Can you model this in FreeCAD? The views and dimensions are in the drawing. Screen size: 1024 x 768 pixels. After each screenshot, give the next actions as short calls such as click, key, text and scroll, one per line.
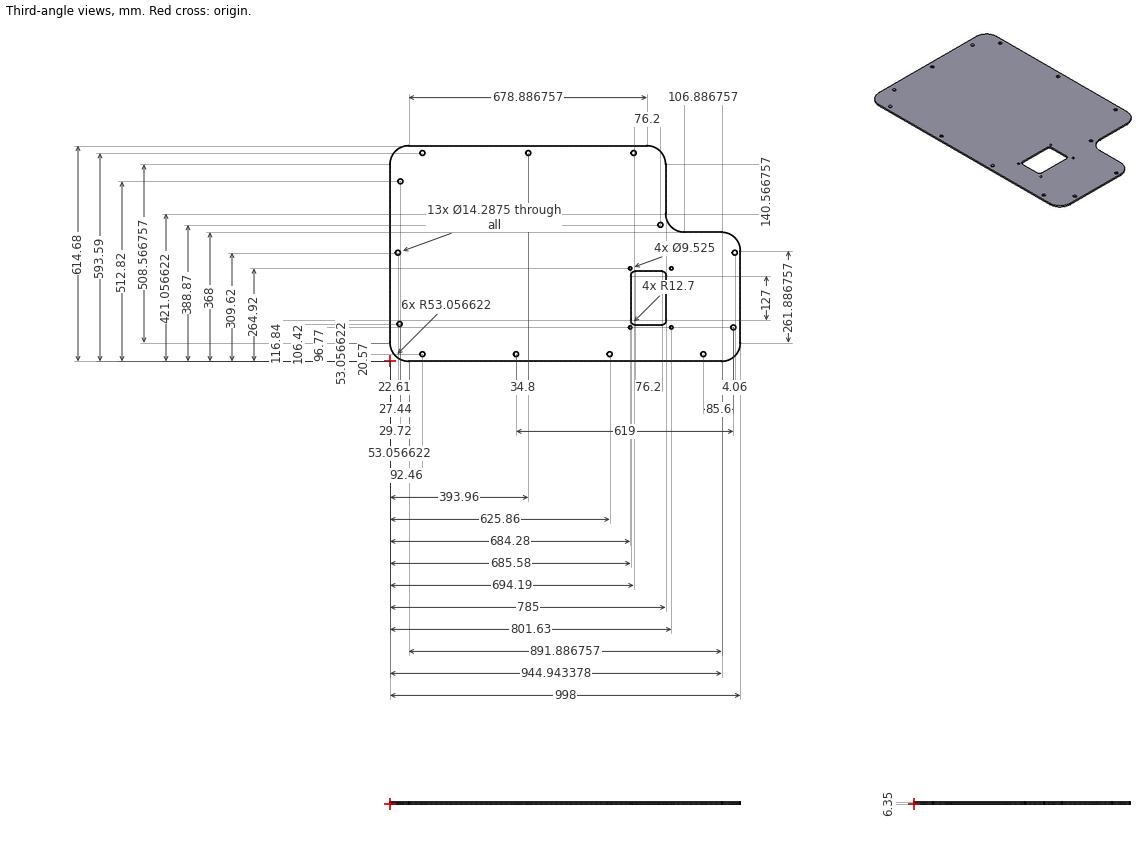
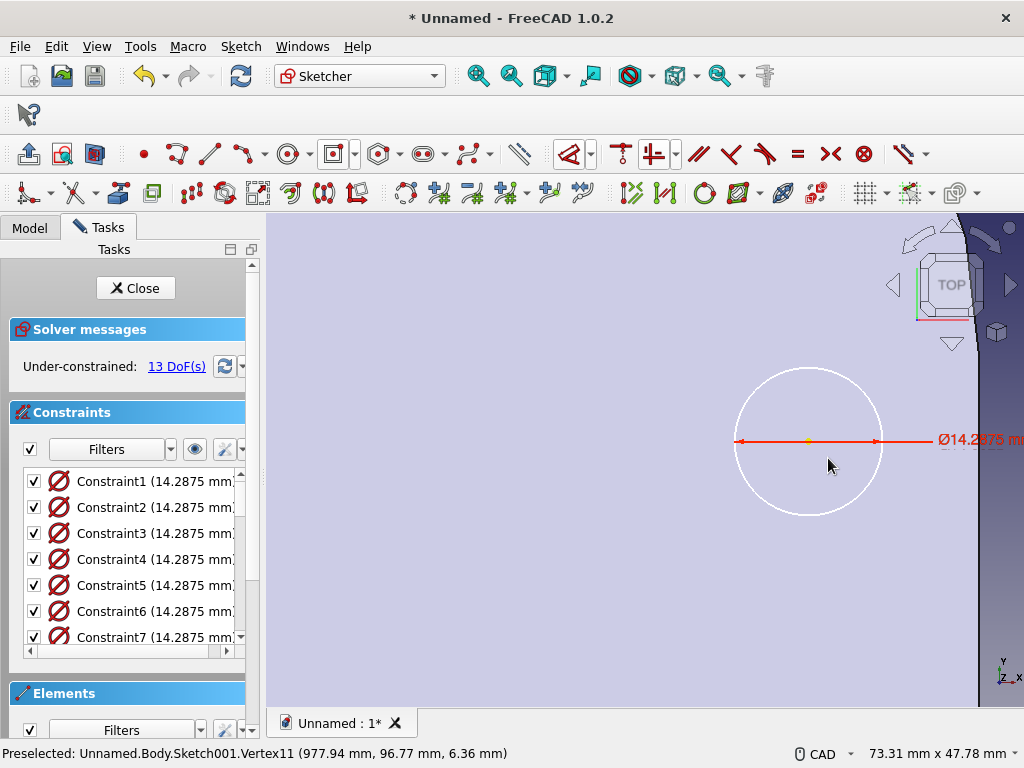
click(809, 442)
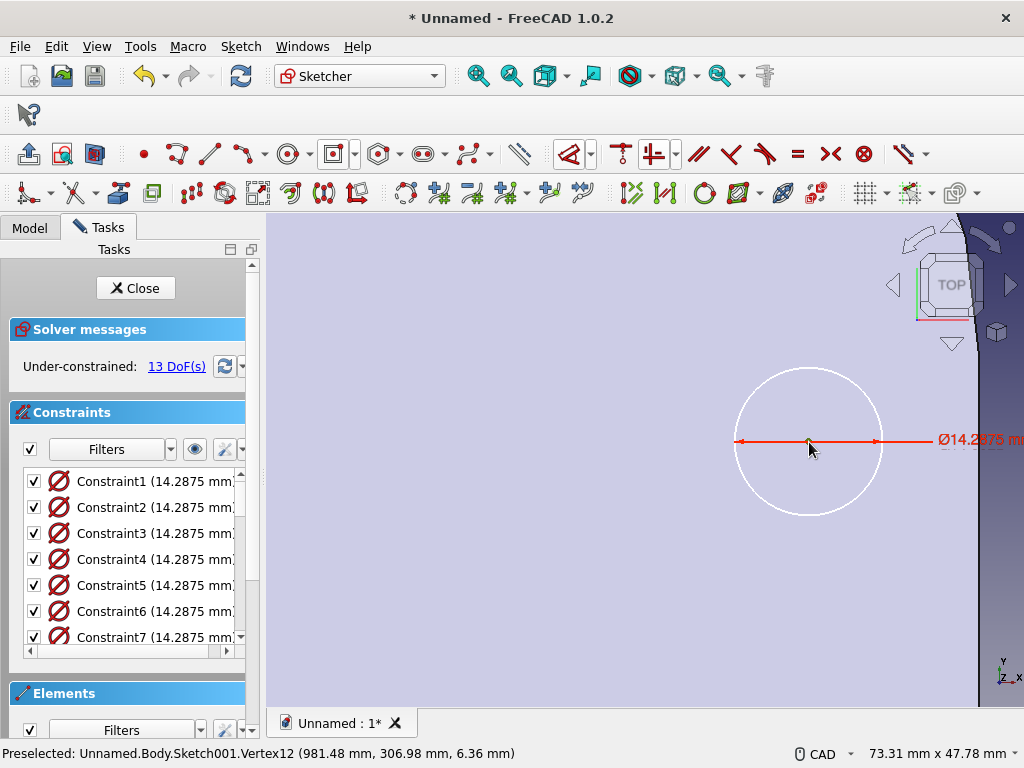
click(590, 154)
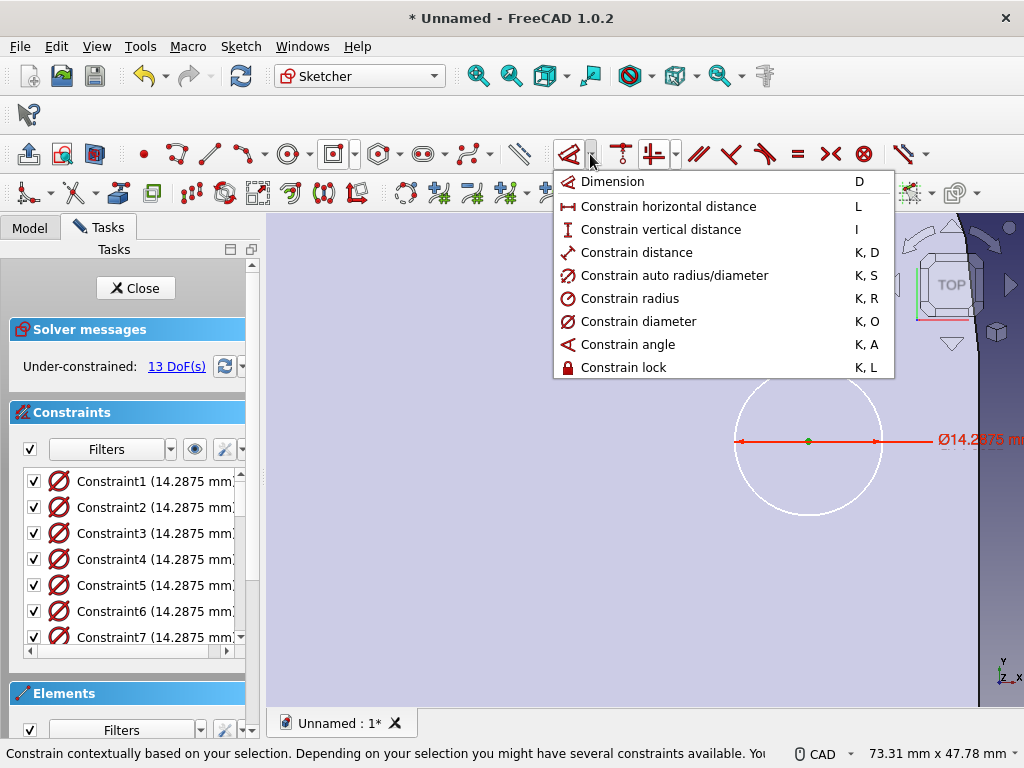
click(724, 206)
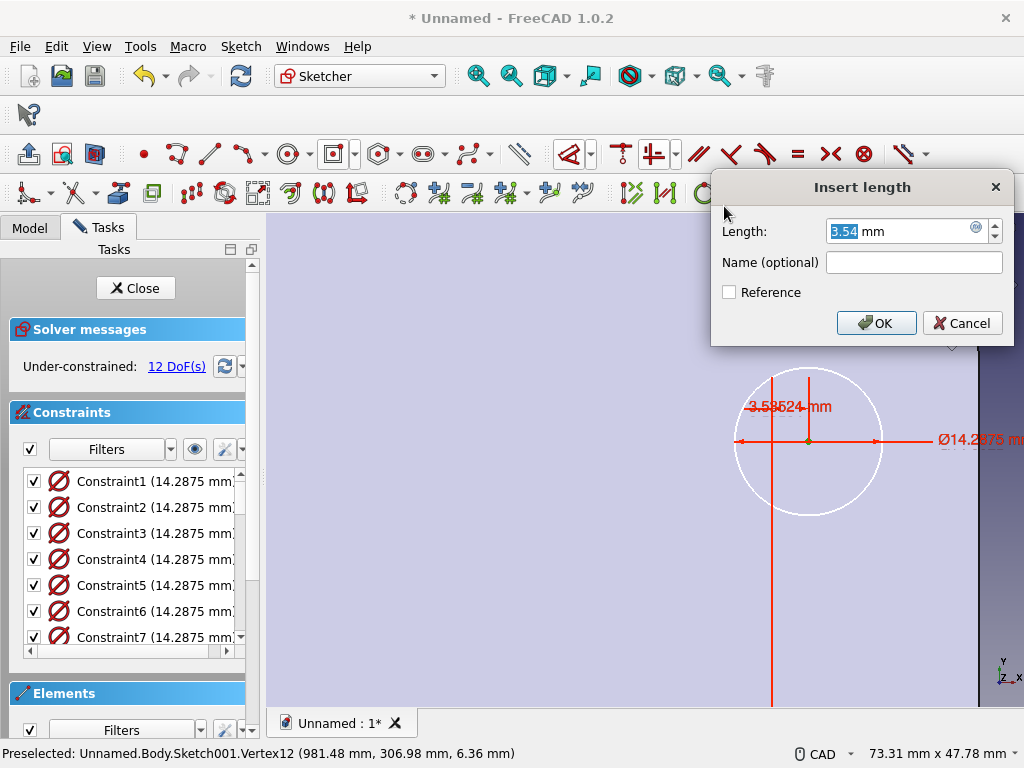
text(4.06)
key(Return)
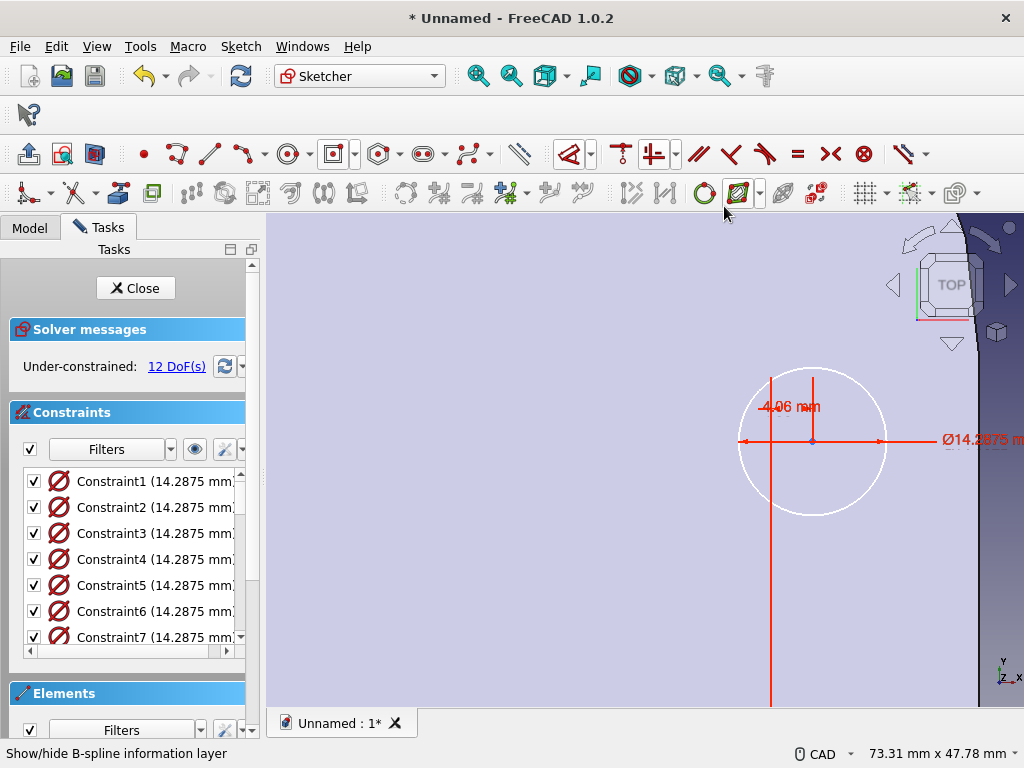
scroll(828, 457, down, 15)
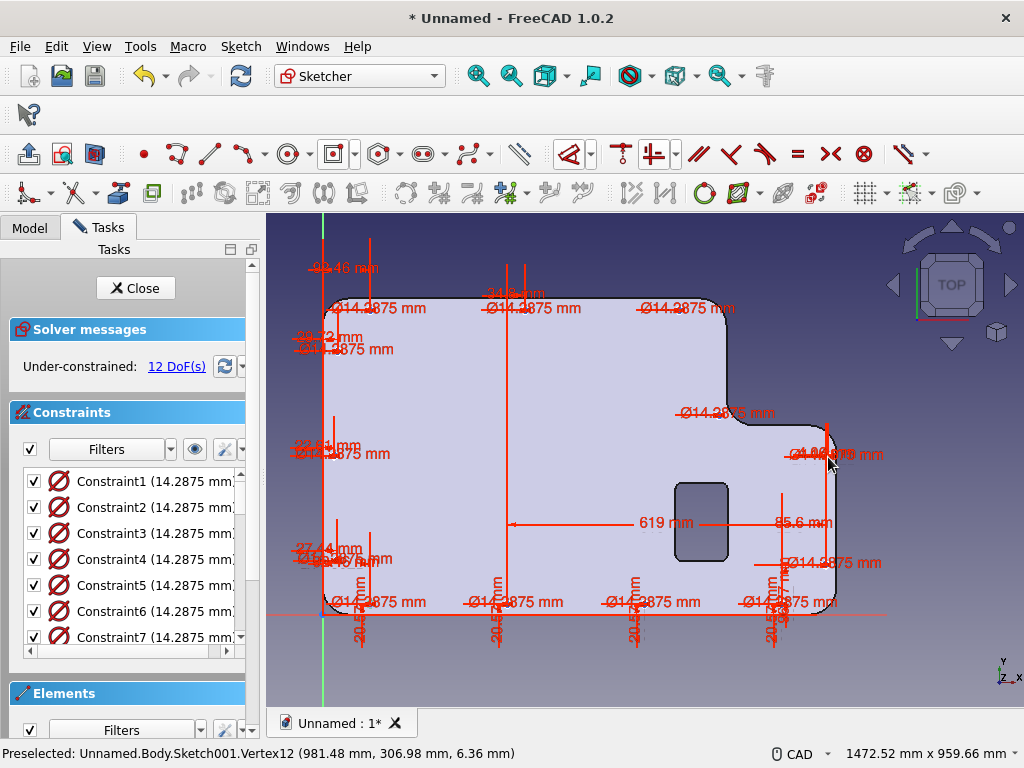
click(679, 310)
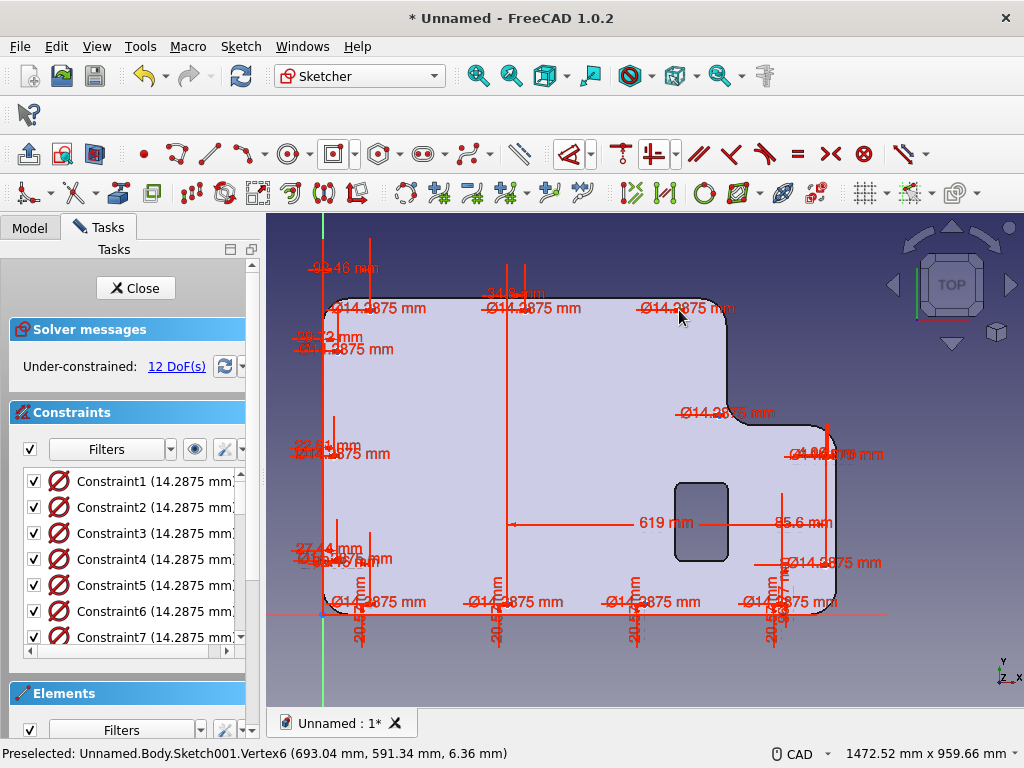
click(719, 415)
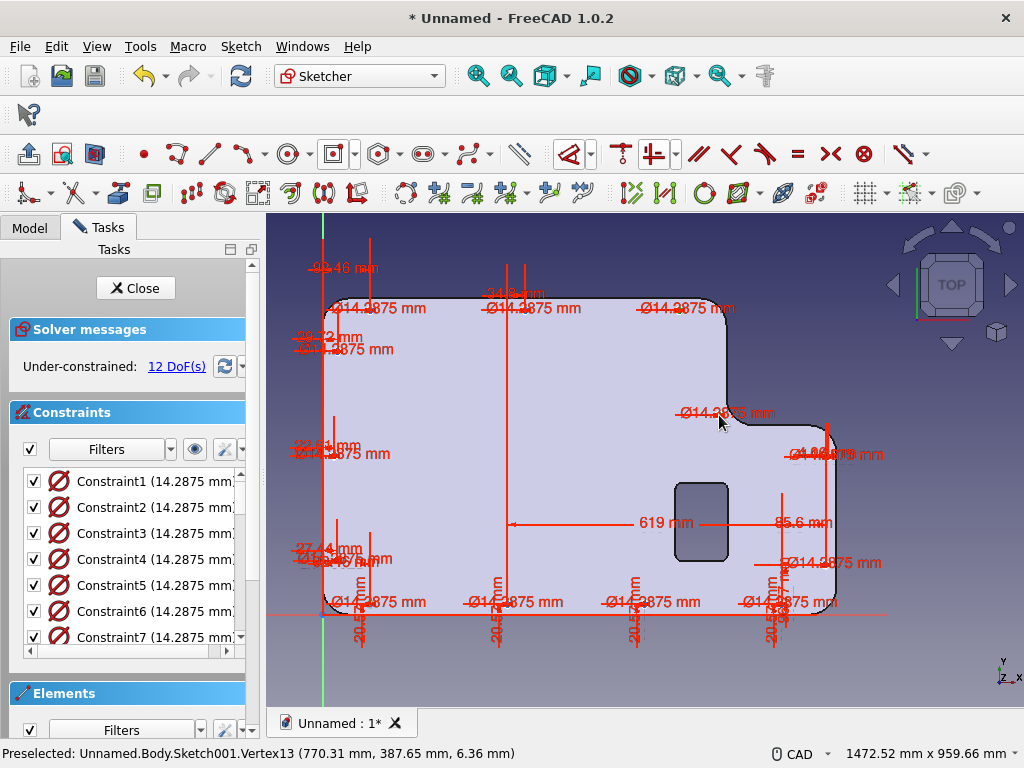
key(l)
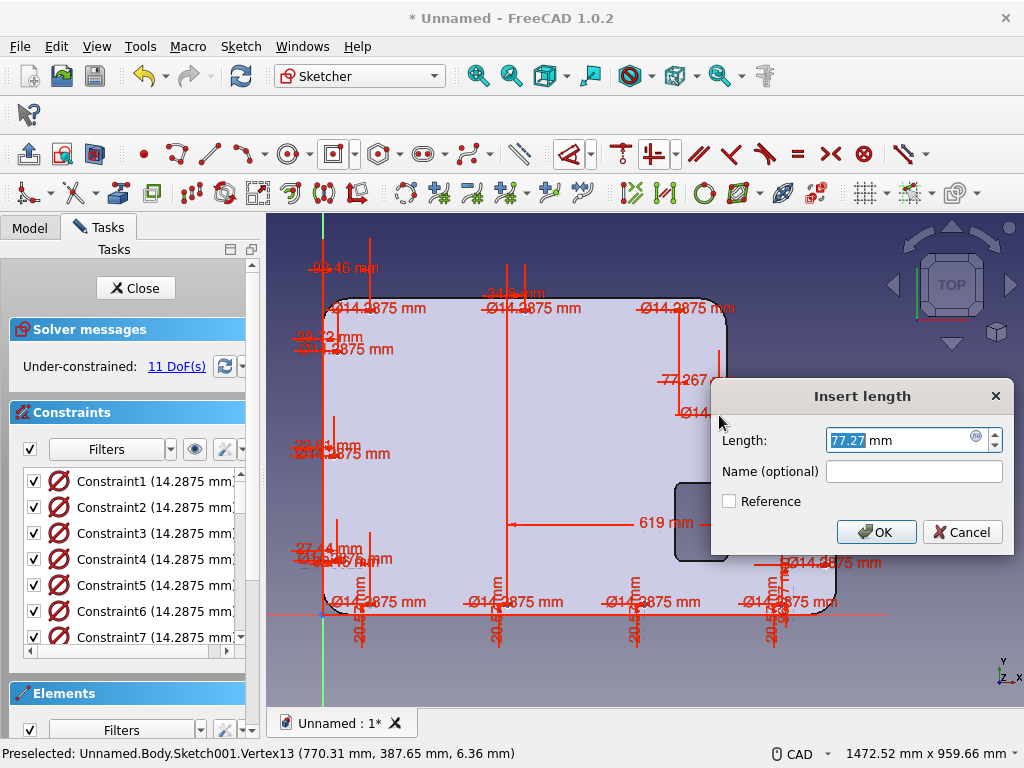
text(76.2)
key(Return)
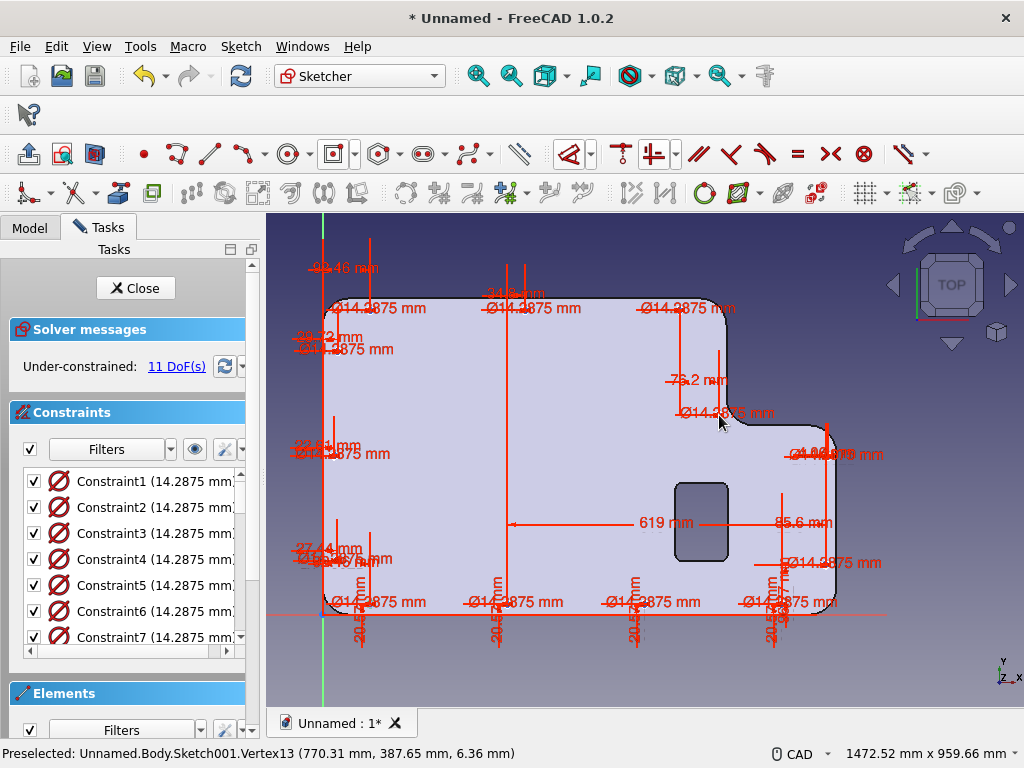
click(334, 456)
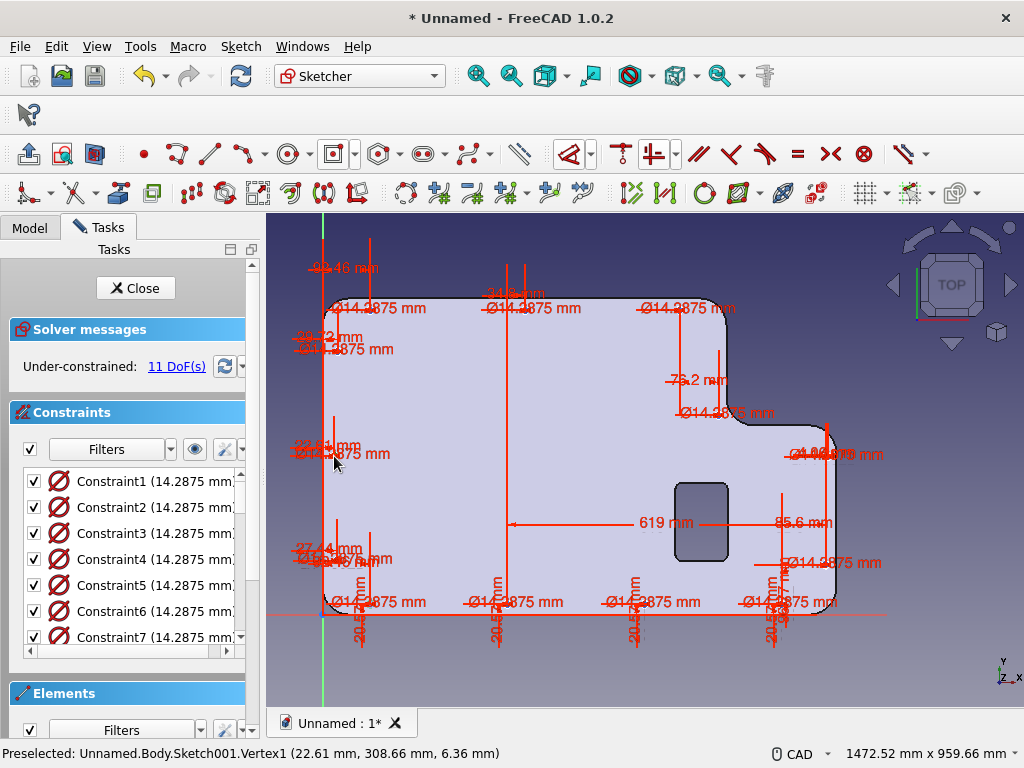
click(590, 154)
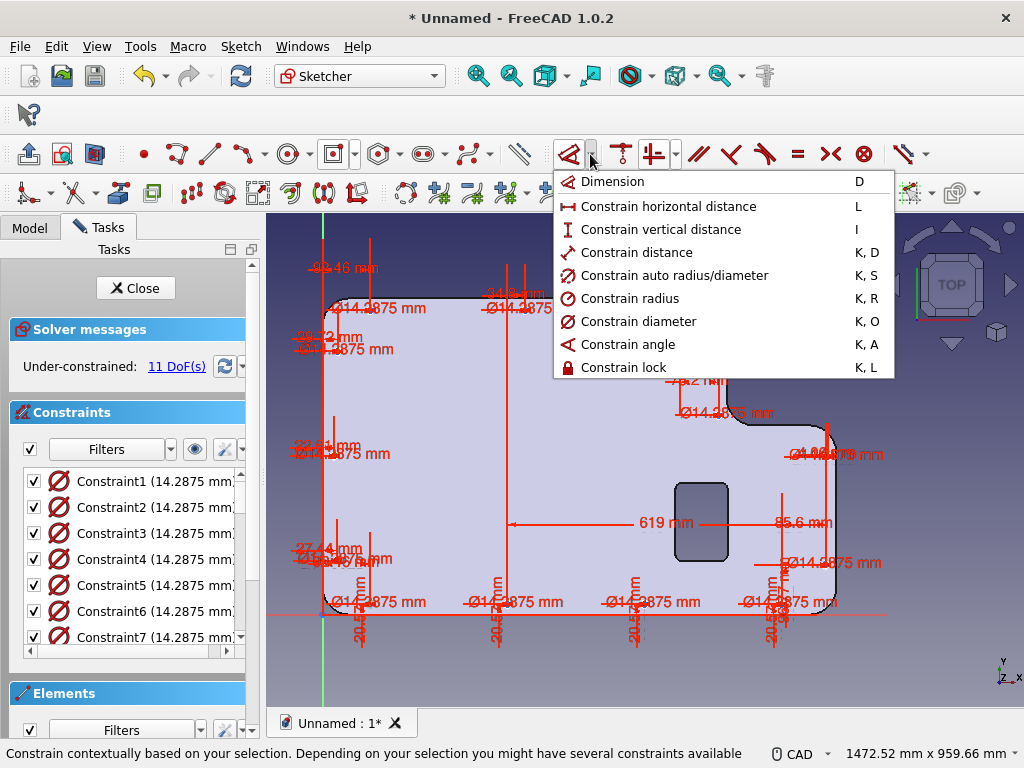
click(724, 230)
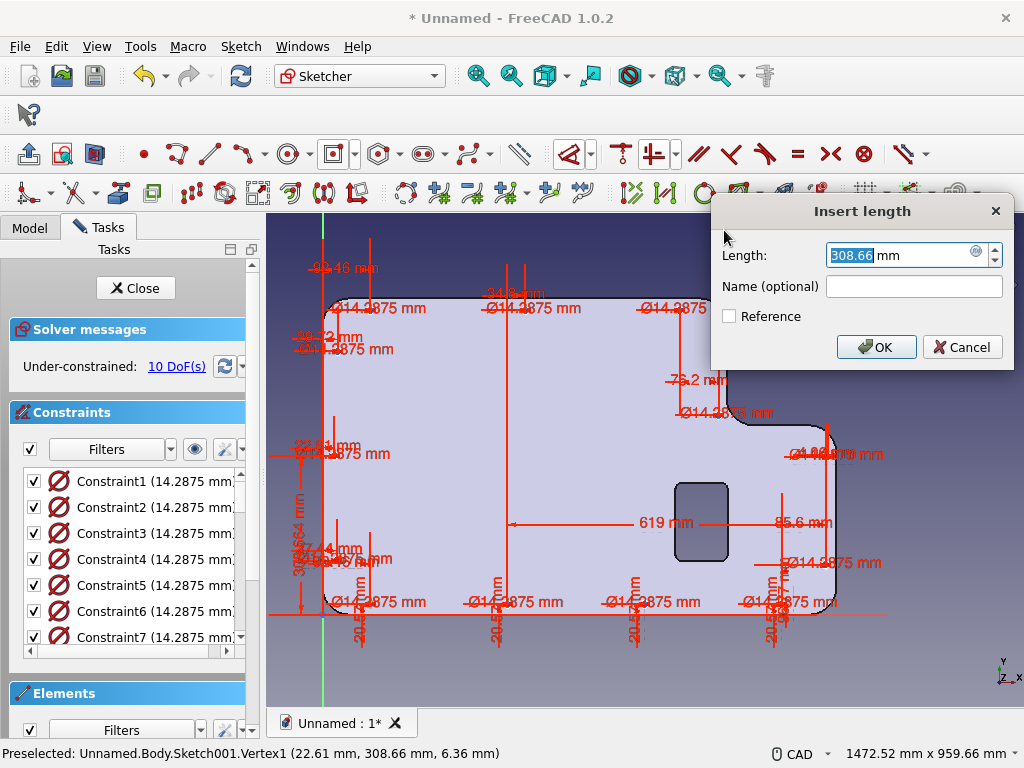
text(309.62)
key(Return)